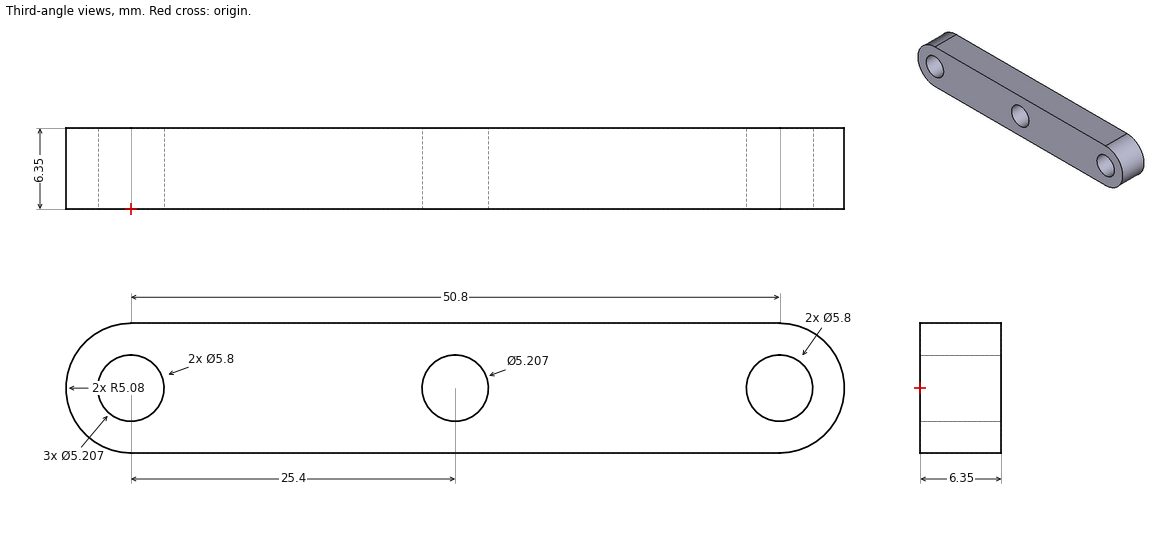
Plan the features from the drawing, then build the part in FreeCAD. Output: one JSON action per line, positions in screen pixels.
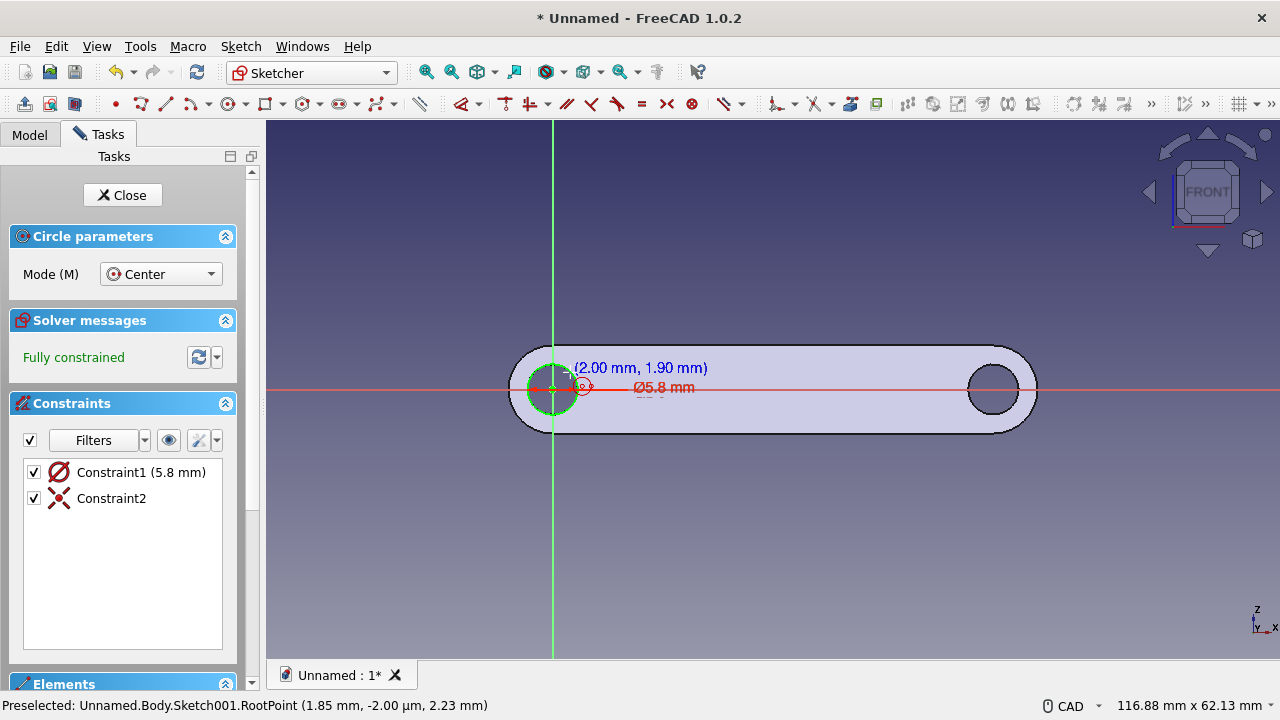
{"action": "left_click", "coordinate": [993, 390]}
{"action": "mouse_move", "coordinate": [1011, 372]}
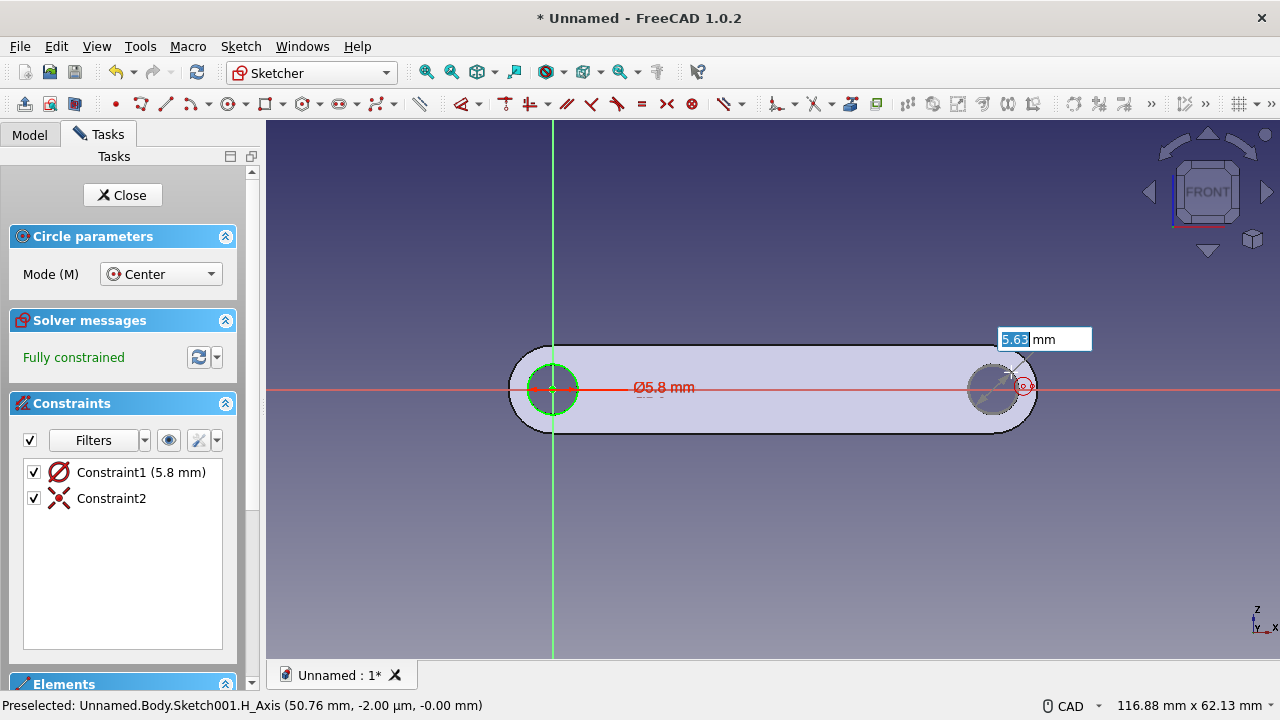
{"action": "type", "text": "5.8"}
{"action": "key", "text": "Return"}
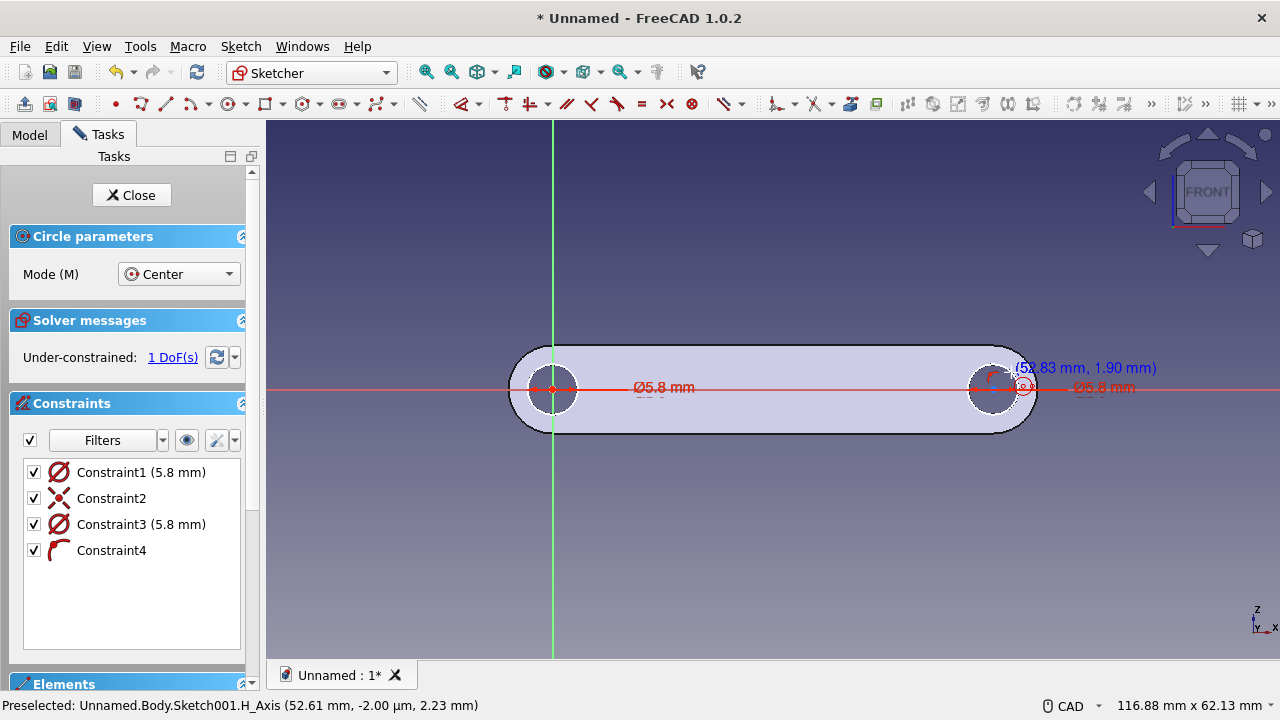
{"action": "left_click", "coordinate": [773, 390]}
{"action": "mouse_move", "coordinate": [789, 374]}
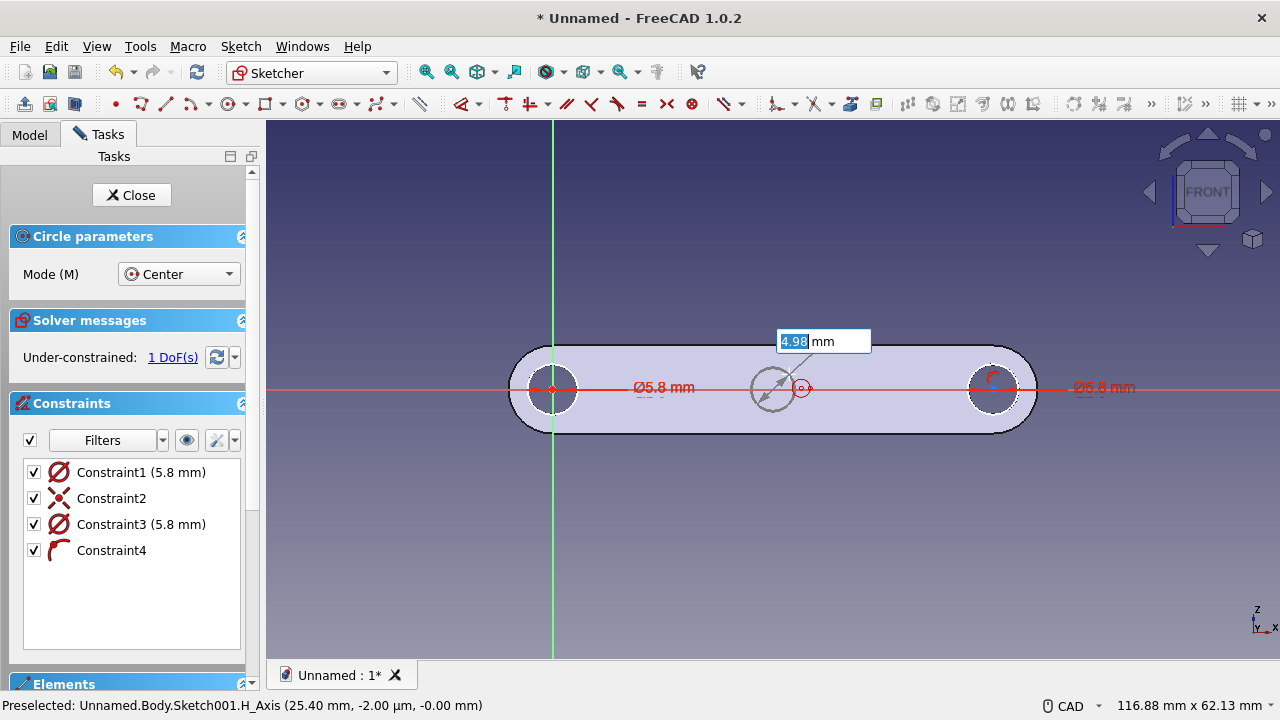
{"action": "type", "text": "5.207"}
{"action": "key", "text": "Return"}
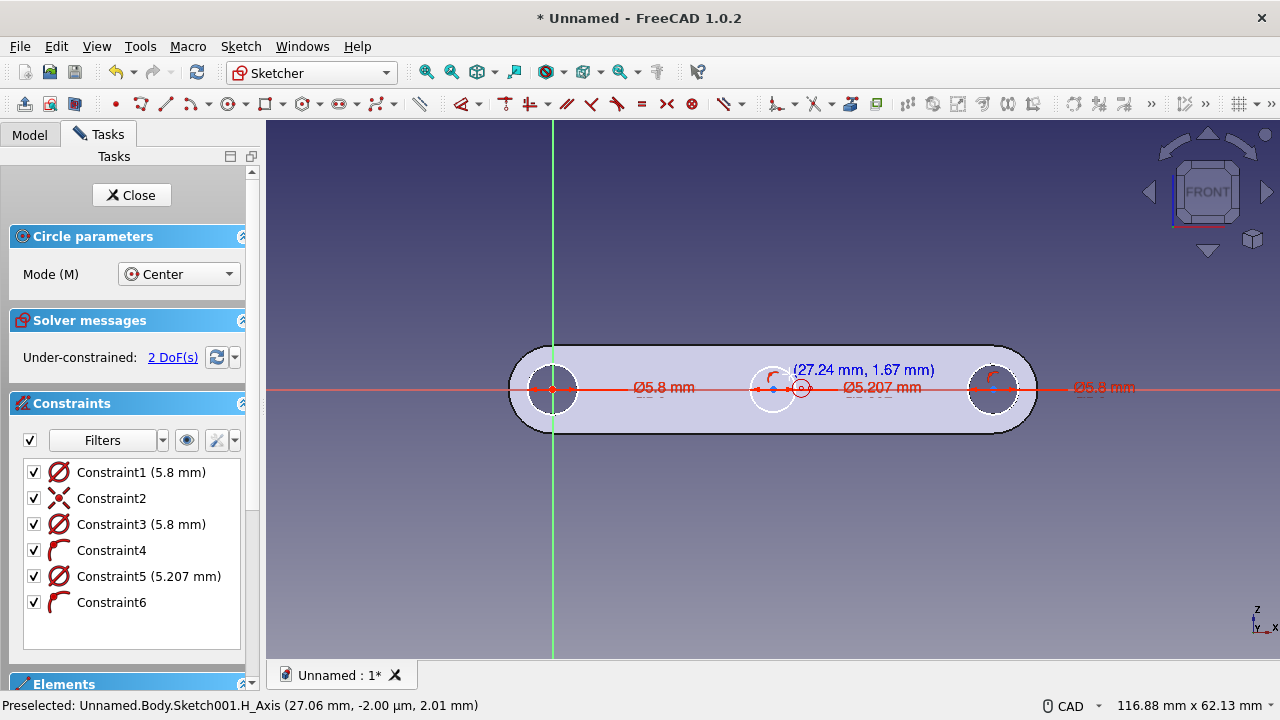
{"action": "left_click", "coordinate": [553, 390]}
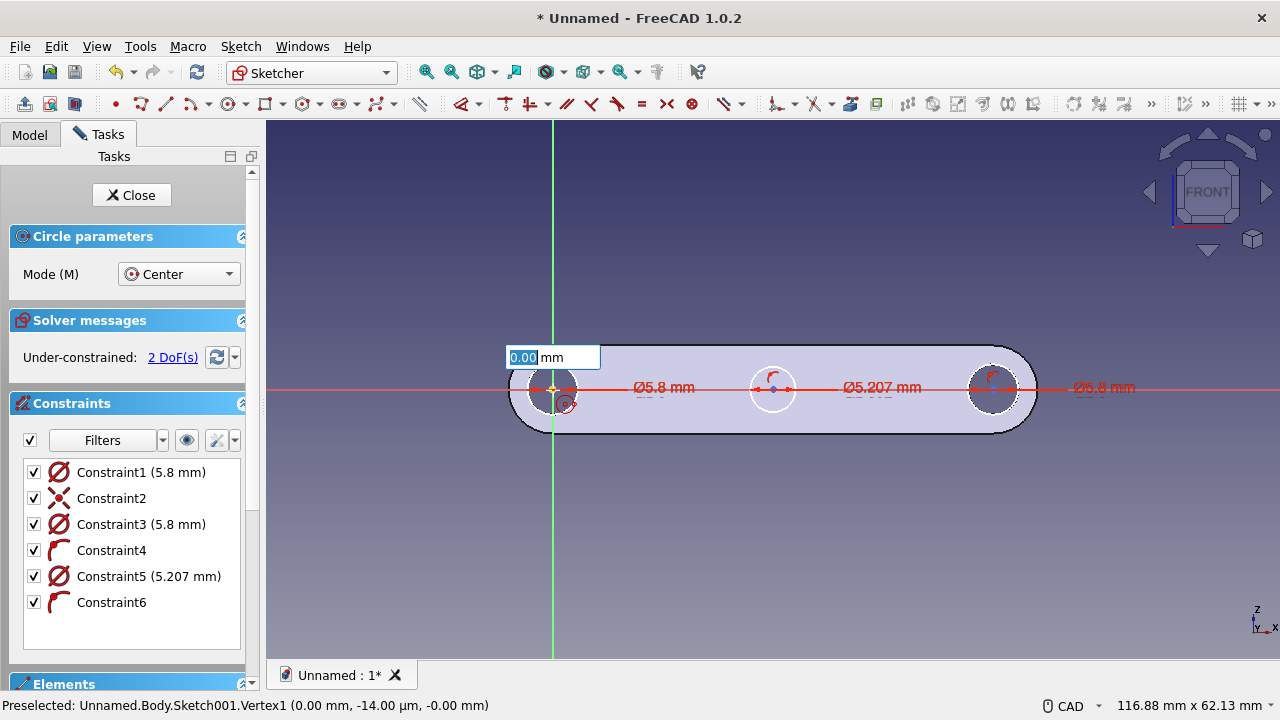
{"action": "scroll", "coordinate": [569, 374], "scroll_direction": "up", "scroll_amount": 10}
{"action": "mouse_move", "coordinate": [564, 367]}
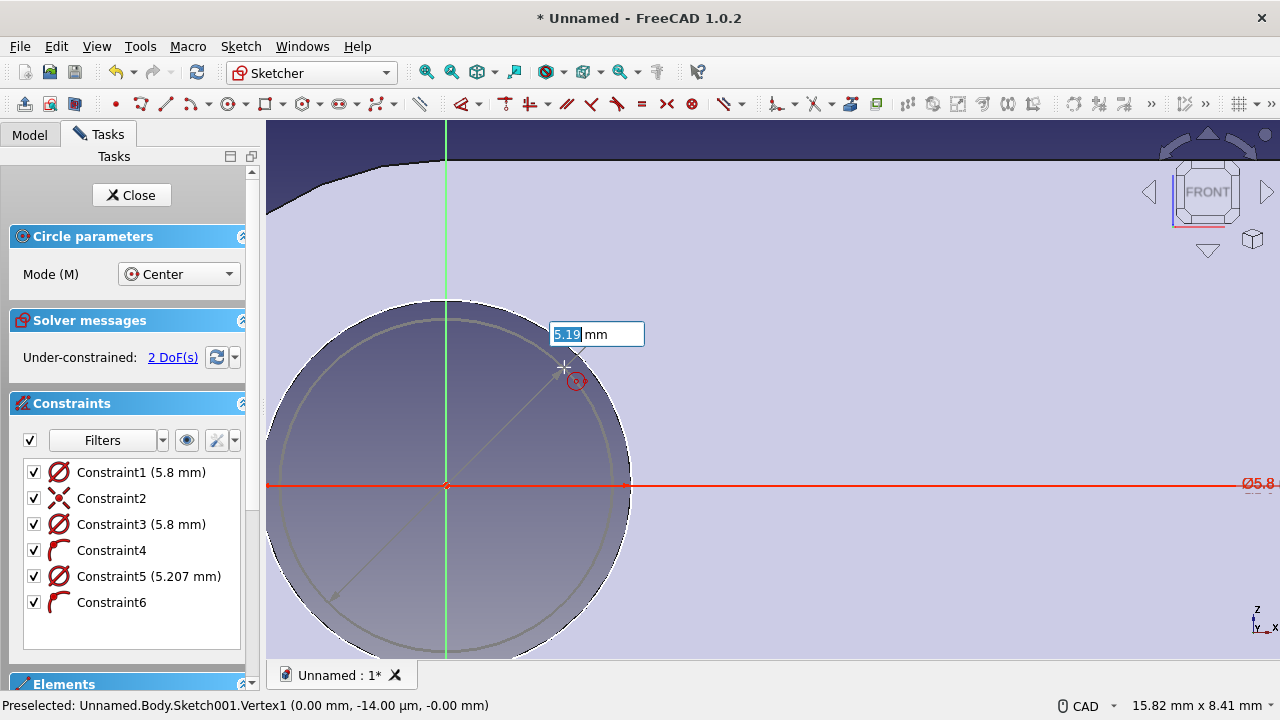
{"action": "type", "text": "5.207"}
{"action": "key", "text": "Return"}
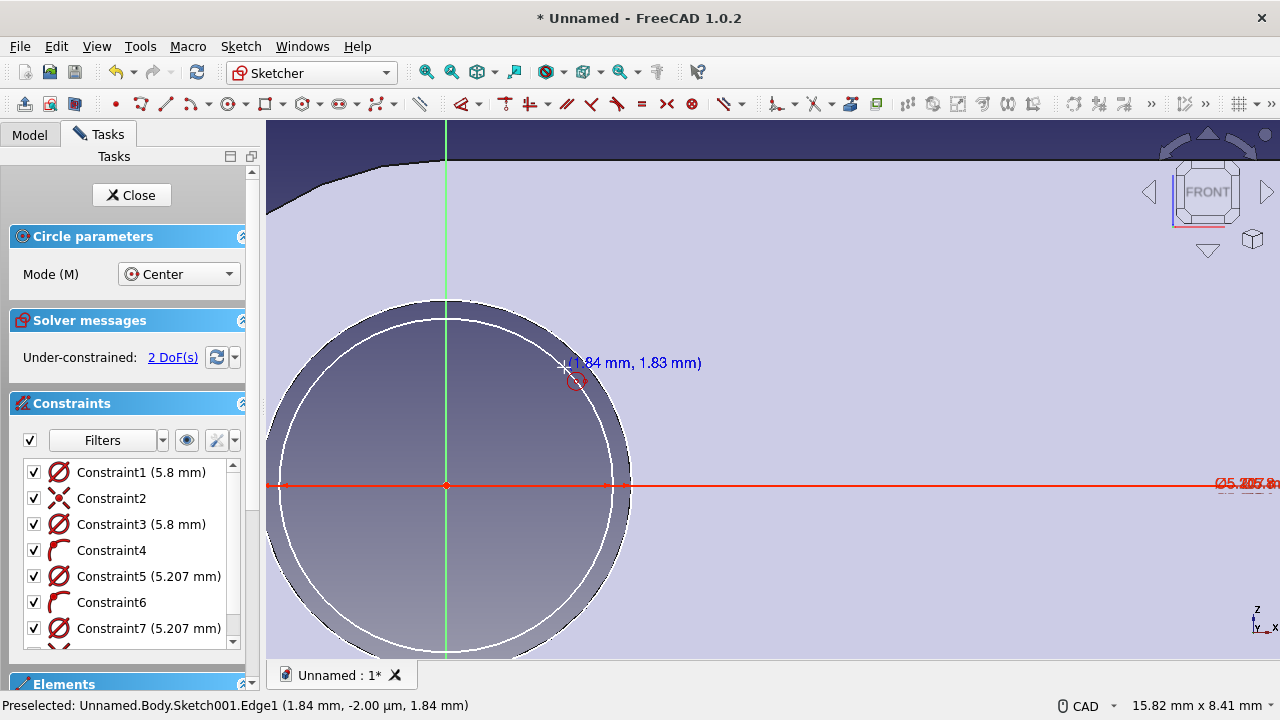
{"action": "scroll", "coordinate": [433, 370], "scroll_direction": "down", "scroll_amount": 9}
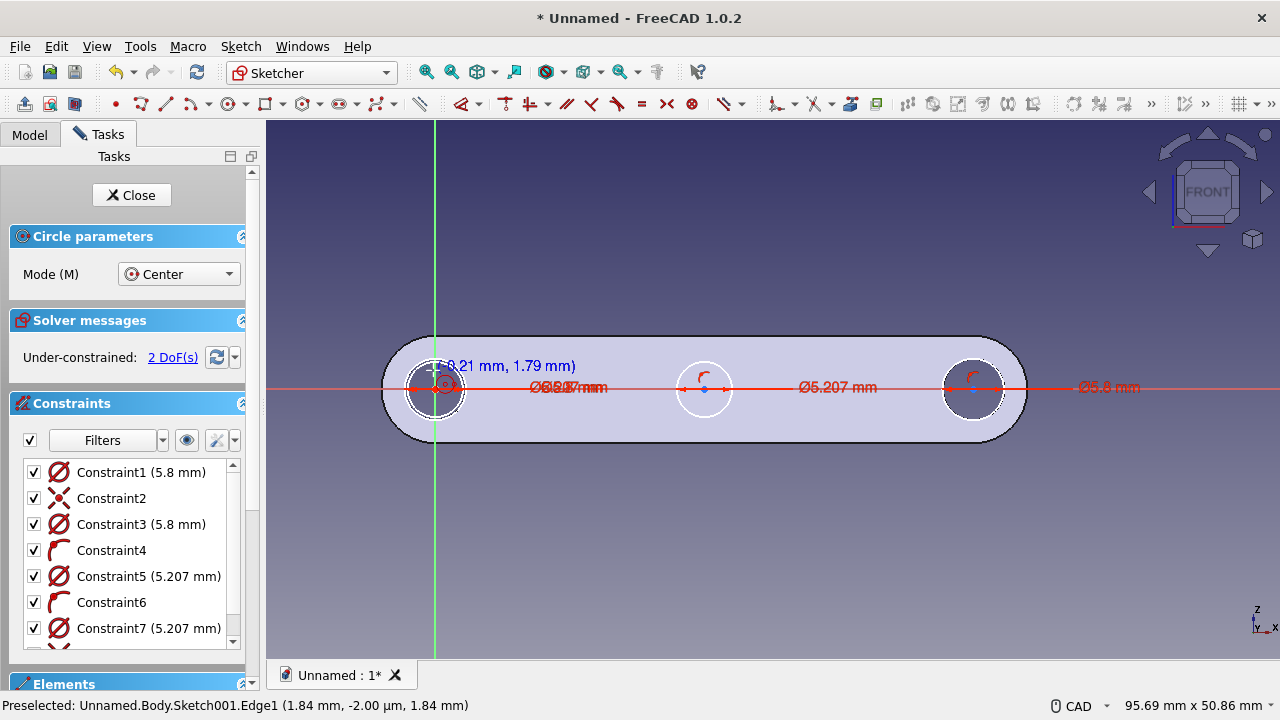
{"action": "left_click", "coordinate": [973, 389]}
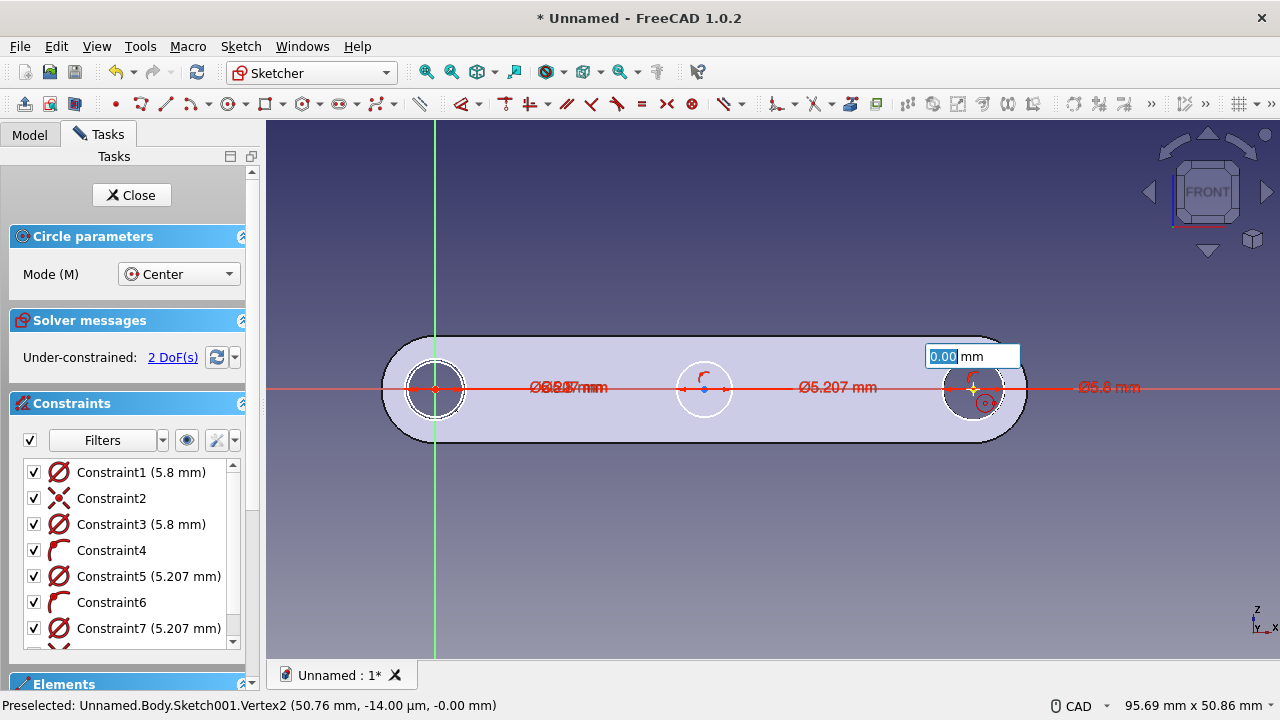
{"action": "scroll", "coordinate": [983, 364], "scroll_direction": "up", "scroll_amount": 9}
{"action": "mouse_move", "coordinate": [980, 359]}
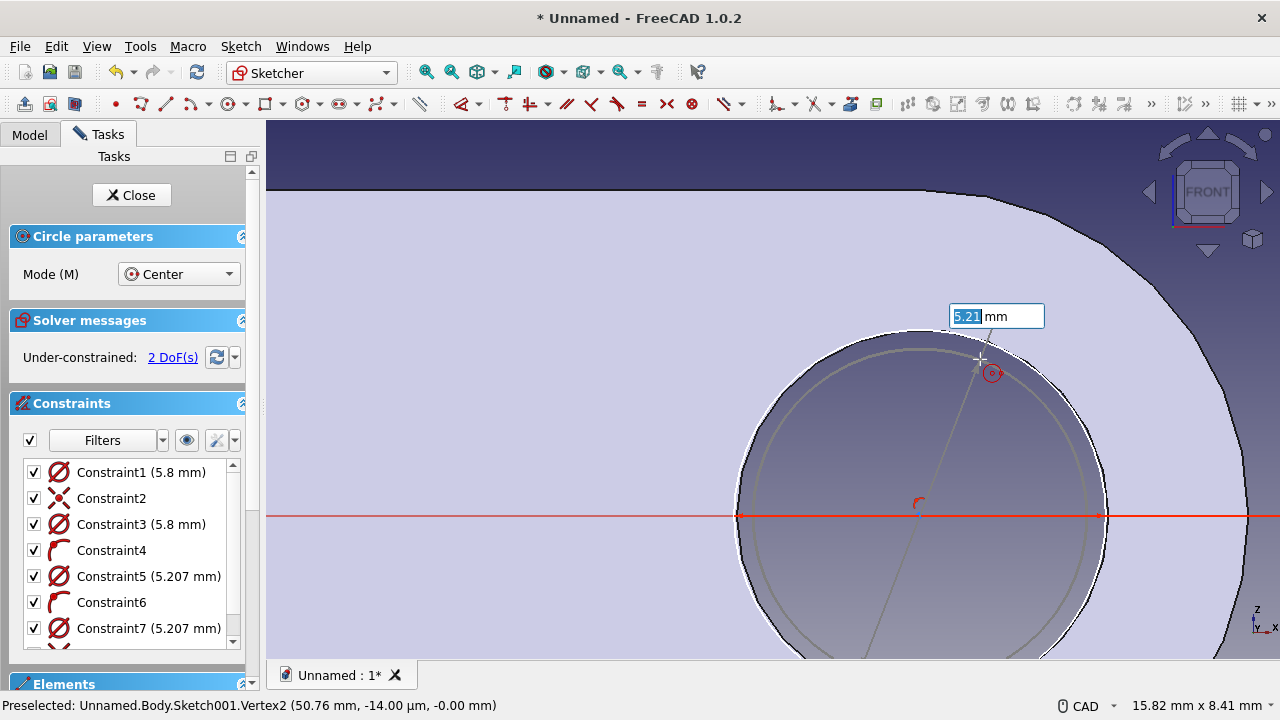
{"action": "type", "text": "5.207"}
{"action": "key", "text": "Return"}
{"action": "key", "text": "Escape"}